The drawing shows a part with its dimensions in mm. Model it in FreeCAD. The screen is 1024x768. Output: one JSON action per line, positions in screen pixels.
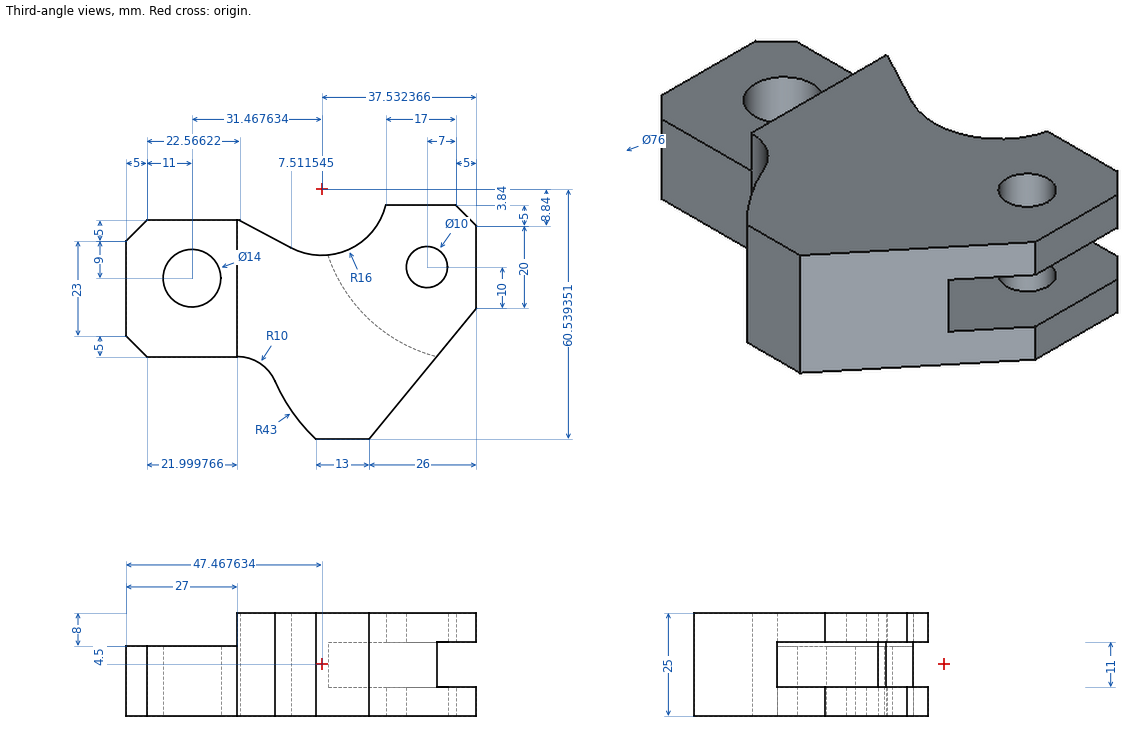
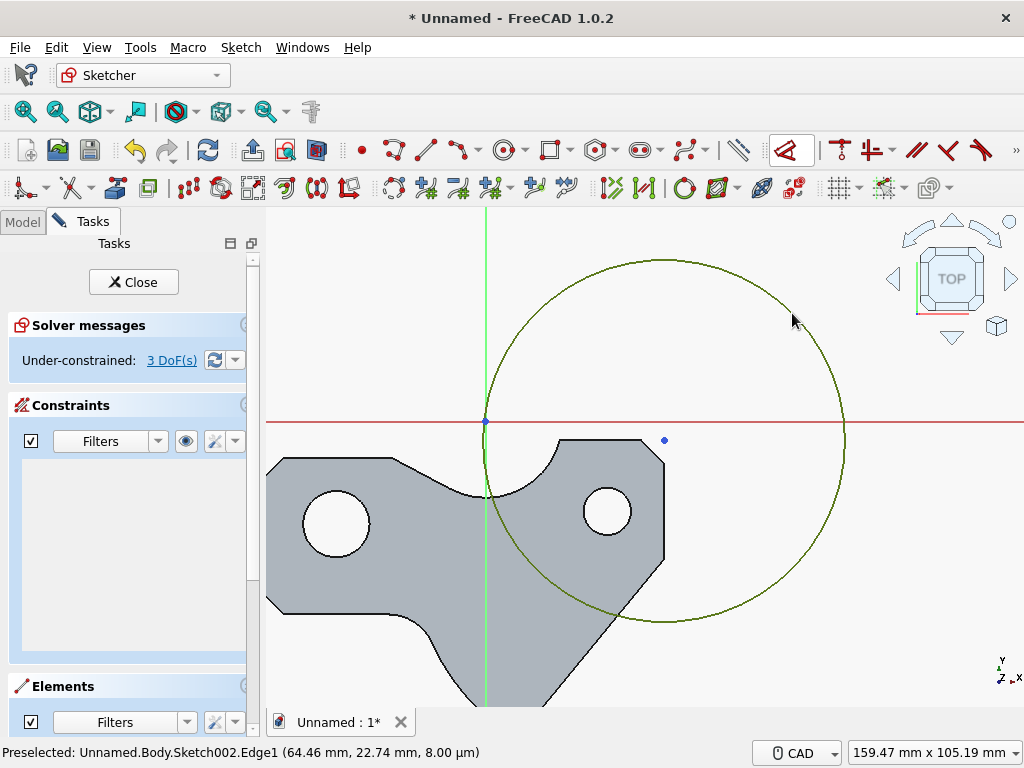
{"action": "left_click", "coordinate": [808, 150]}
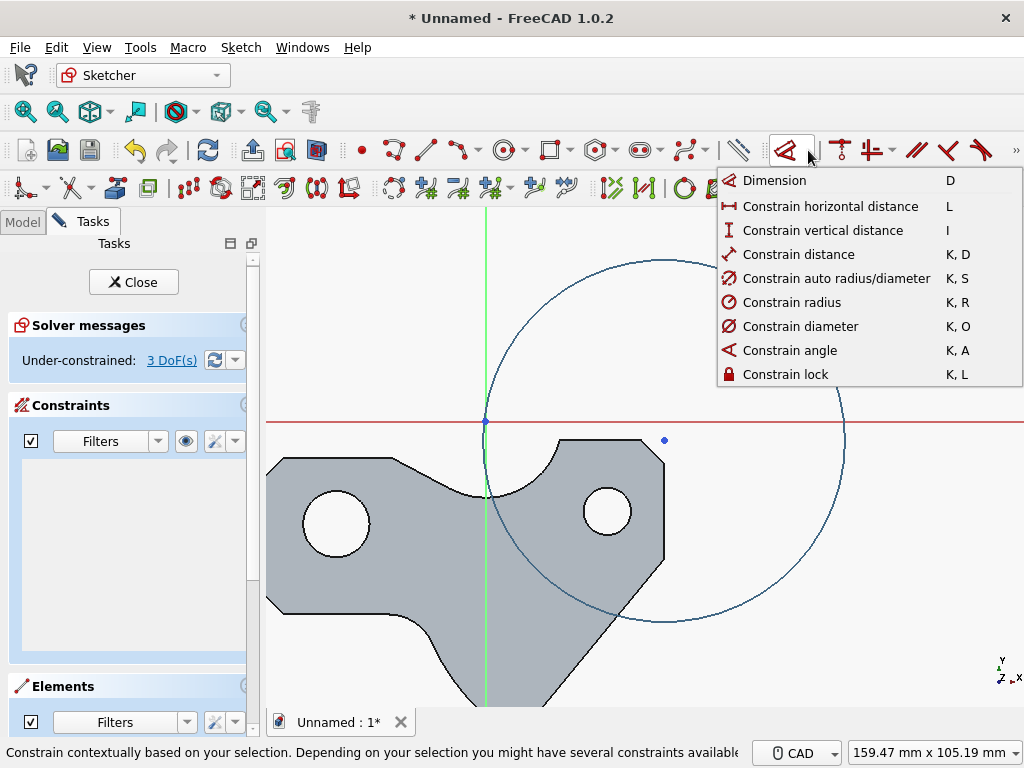
{"action": "left_click", "coordinate": [870, 326]}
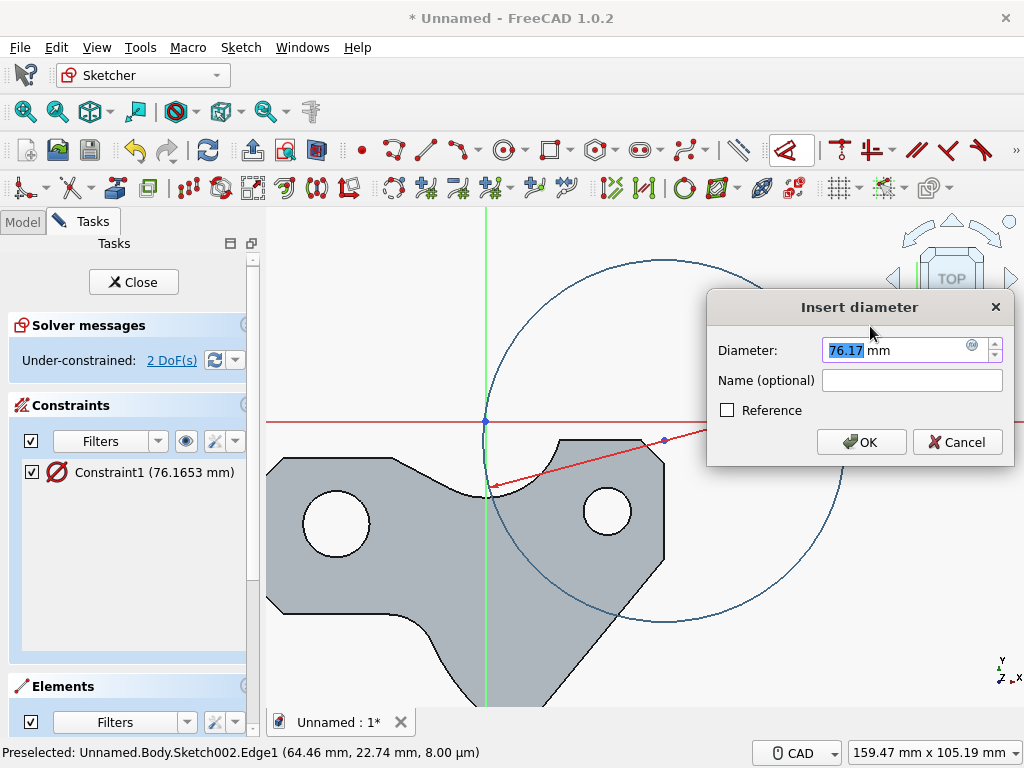
{"action": "type", "text": "76"}
{"action": "key", "text": "Return"}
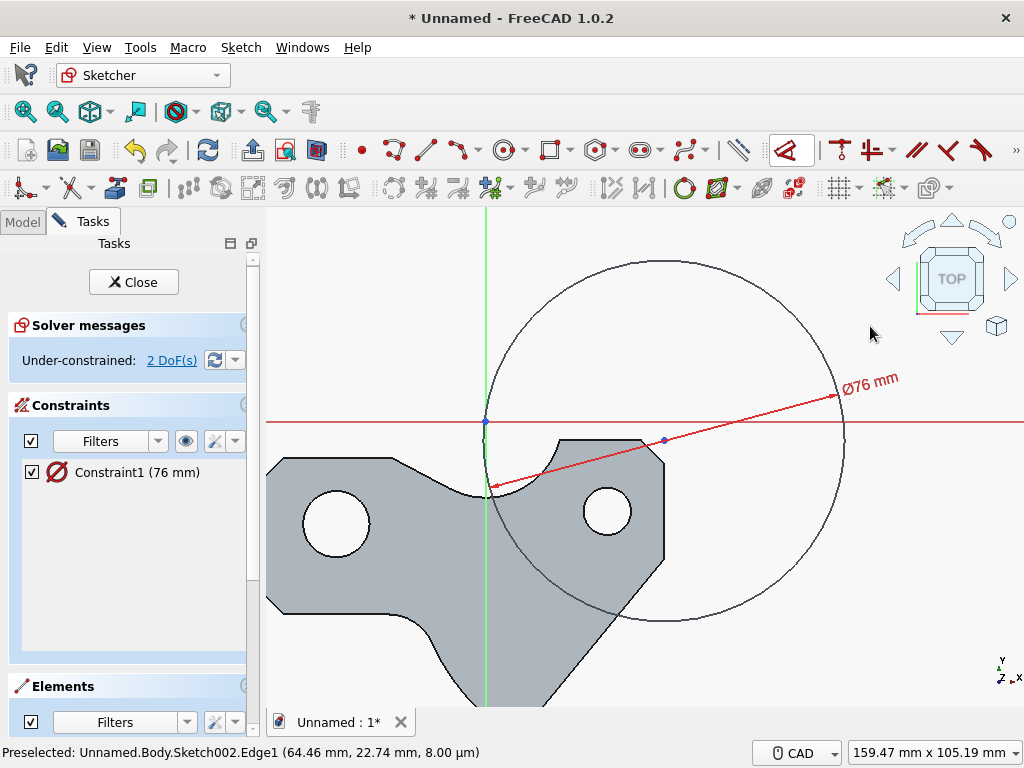
{"action": "scroll", "coordinate": [664, 441], "scroll_direction": "up", "scroll_amount": 4}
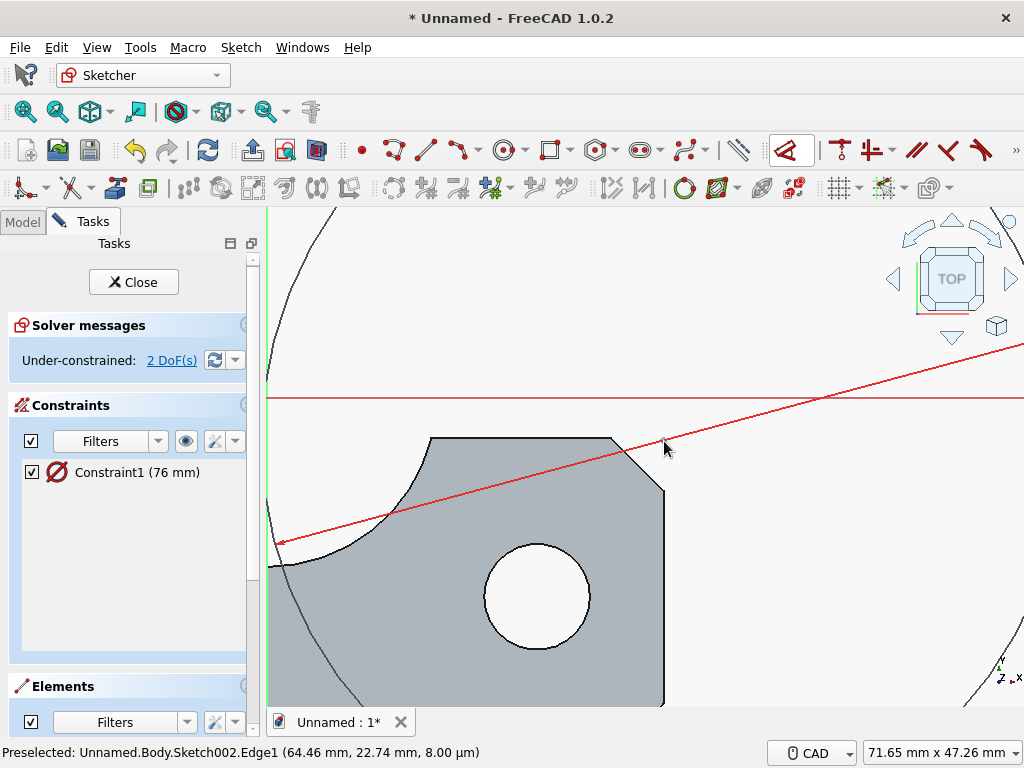
{"action": "left_click", "coordinate": [663, 440]}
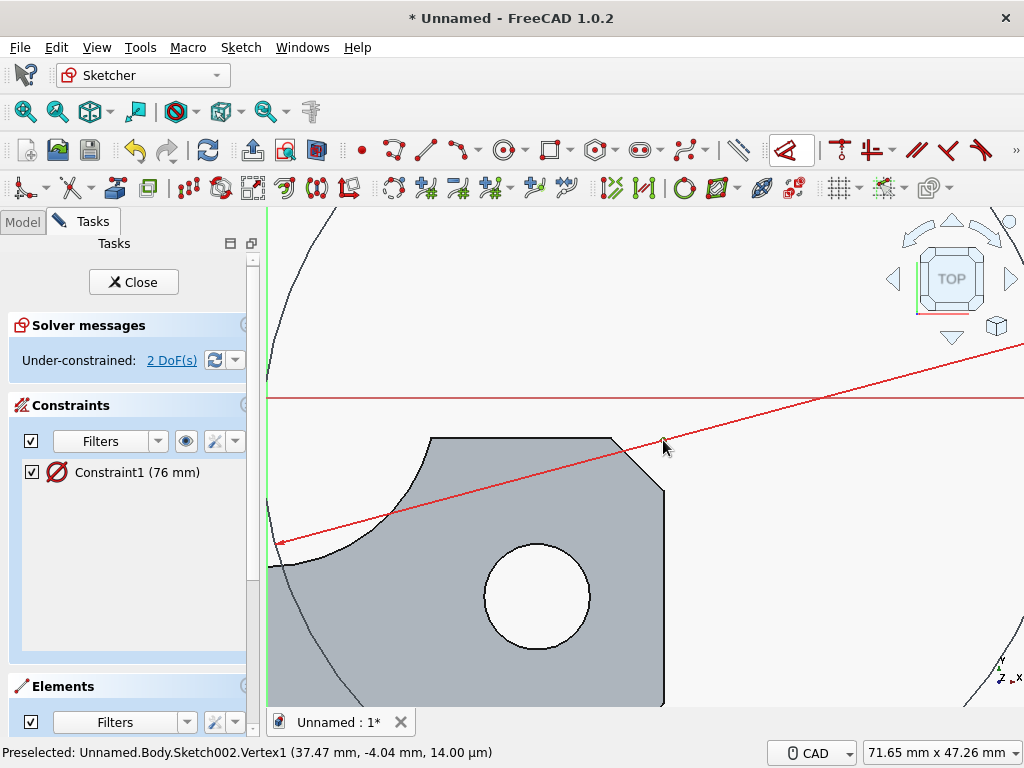
{"action": "key", "text": "i"}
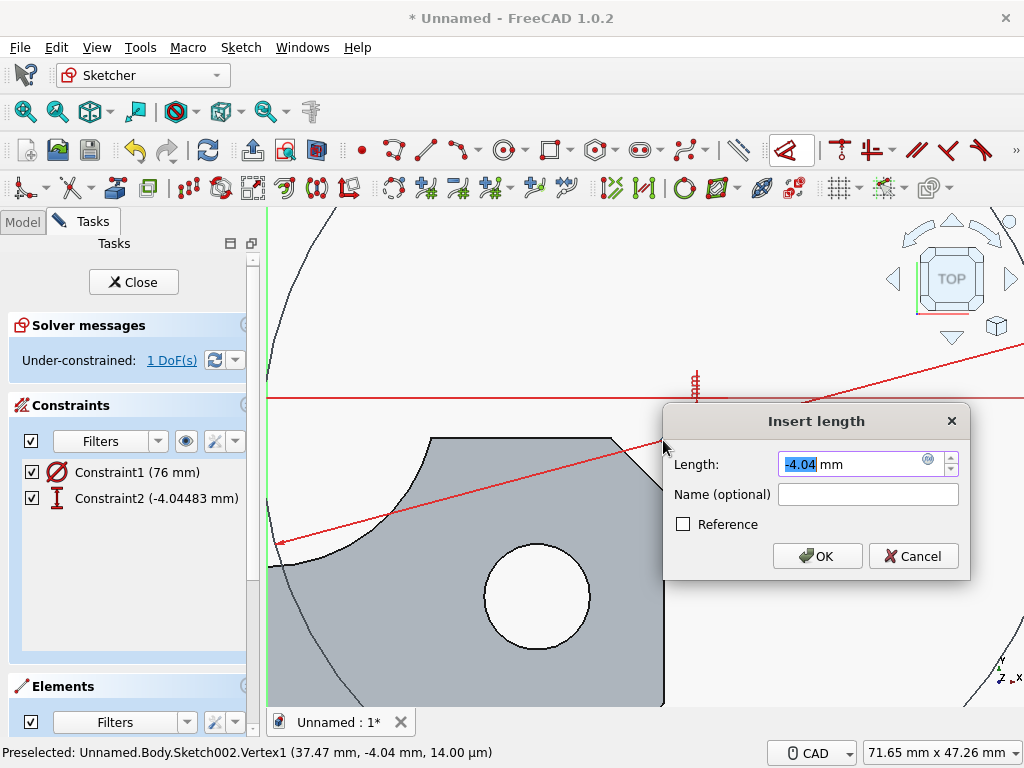
{"action": "type", "text": "-3.84"}
{"action": "key", "text": "Return"}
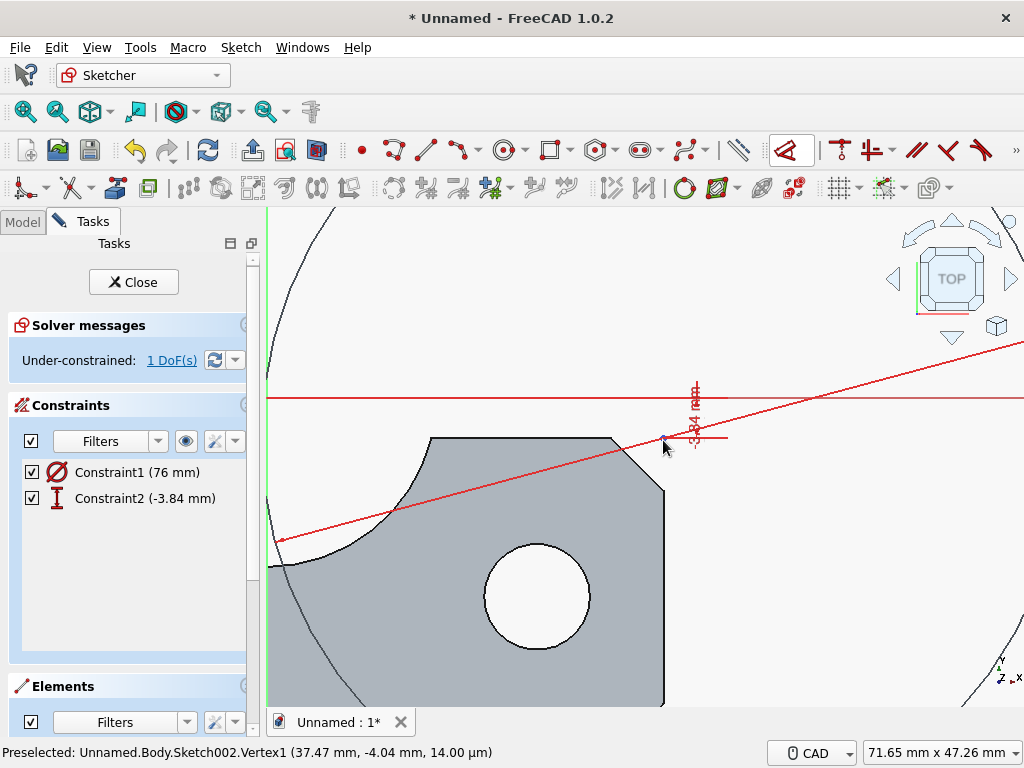
{"action": "left_click", "coordinate": [663, 438]}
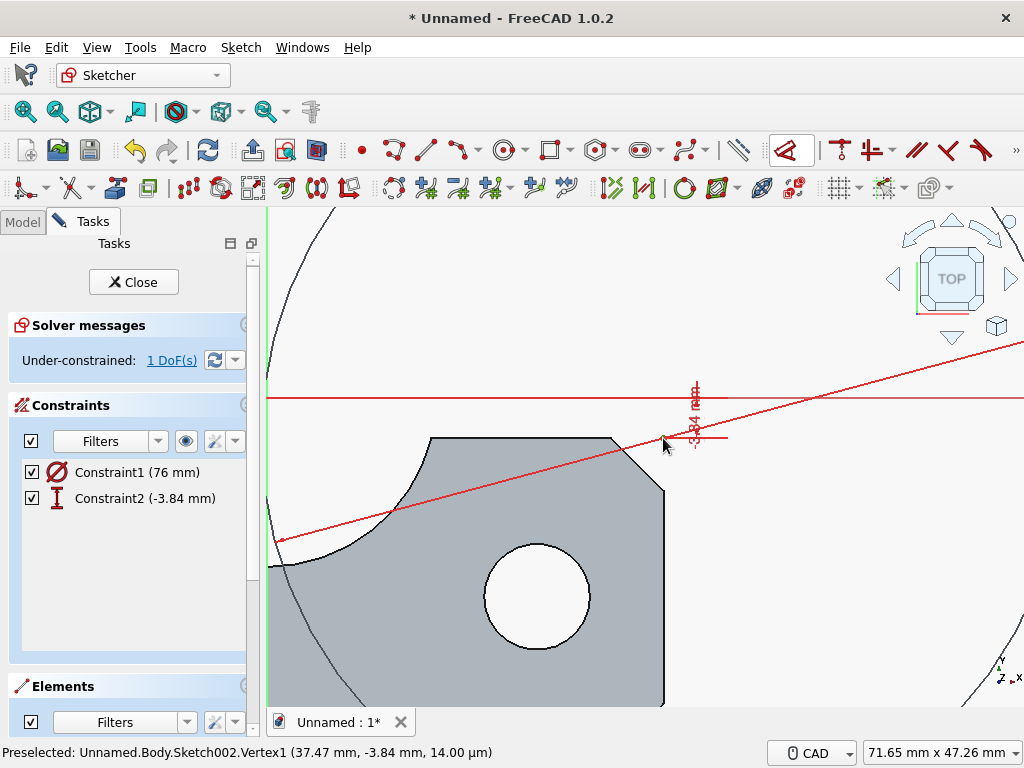
{"action": "key", "text": "l"}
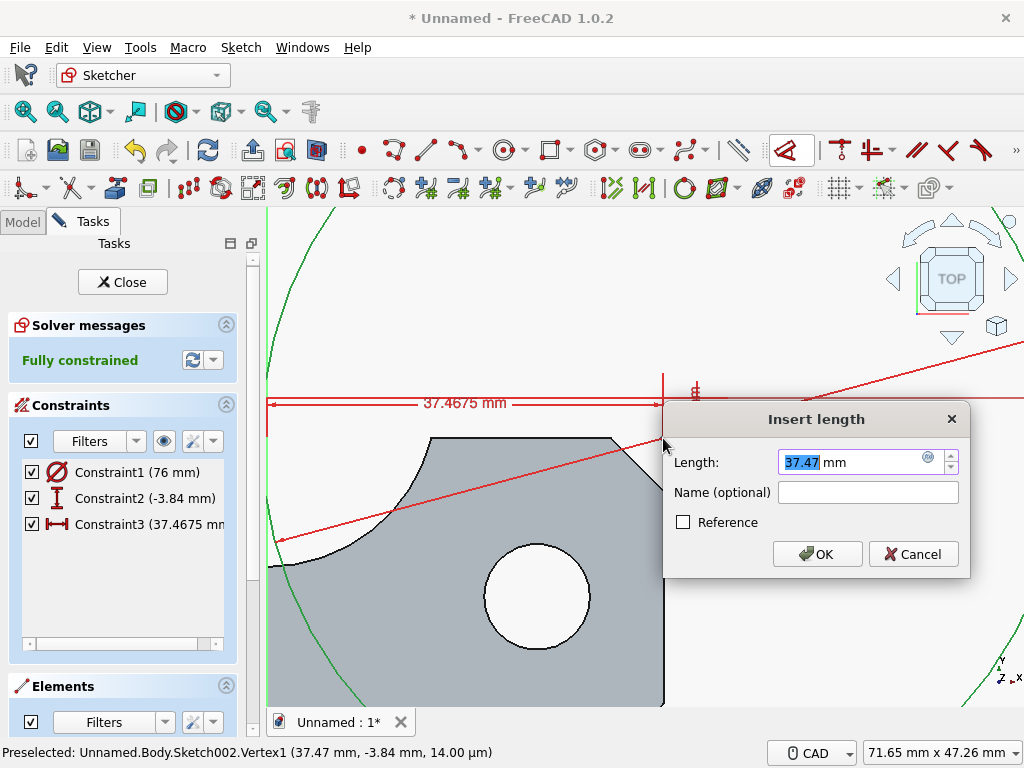
{"action": "type", "text": "37.532366"}
{"action": "key", "text": "Return"}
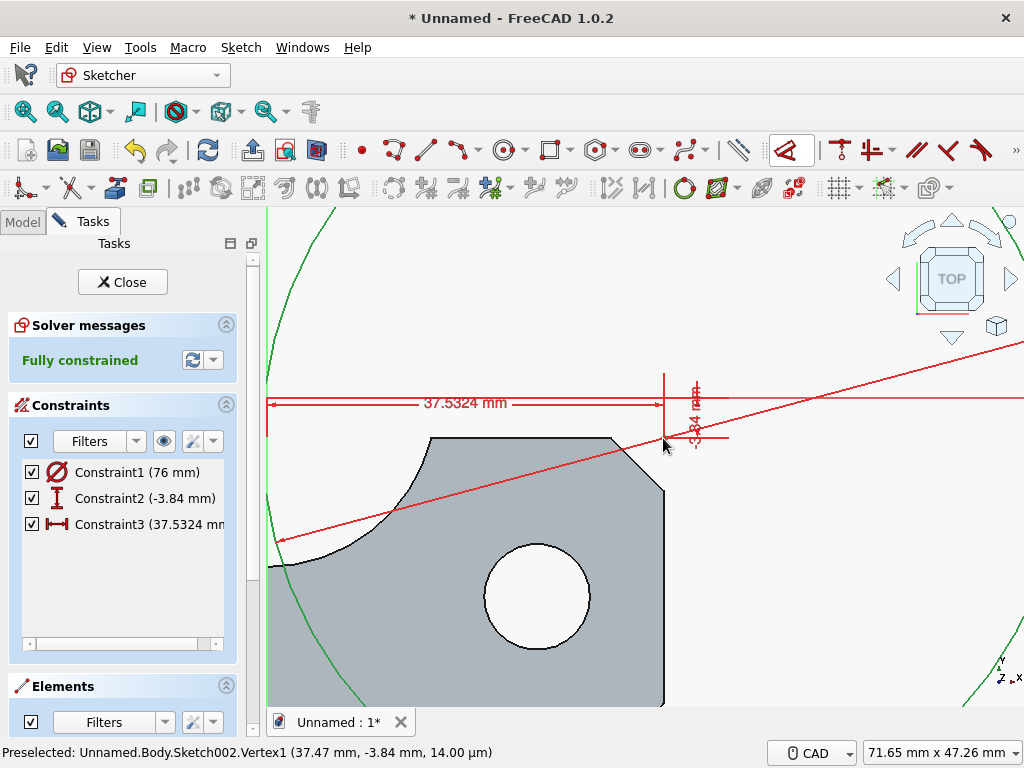
{"action": "left_click", "coordinate": [123, 282]}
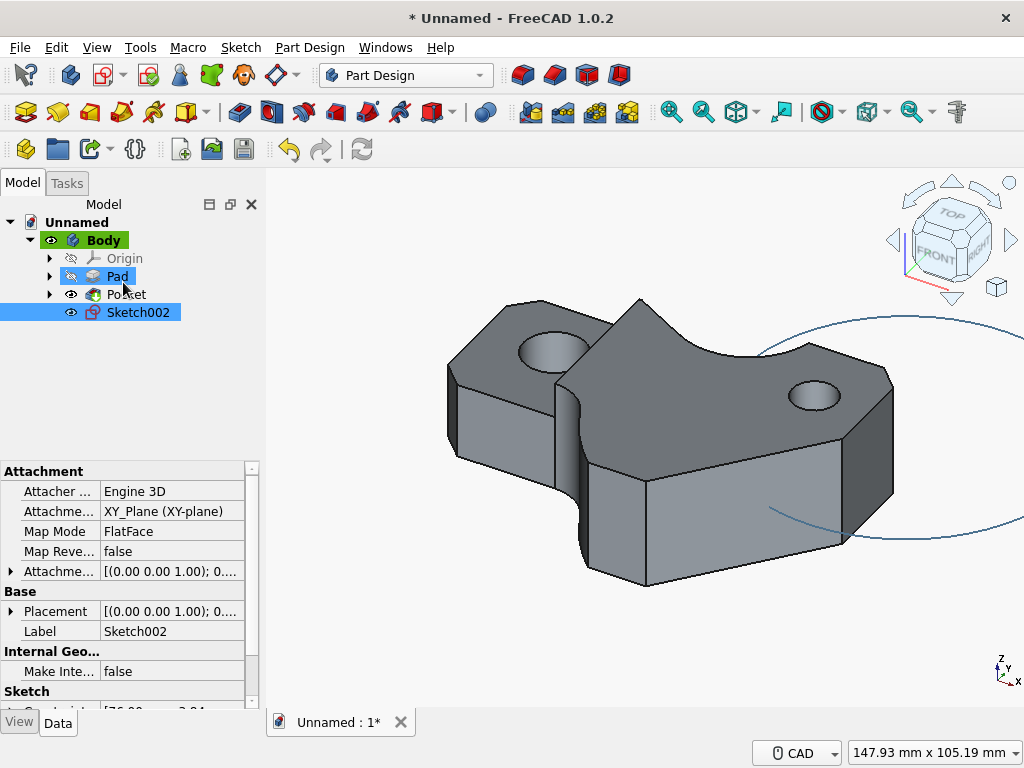
{"action": "left_click", "coordinate": [240, 112]}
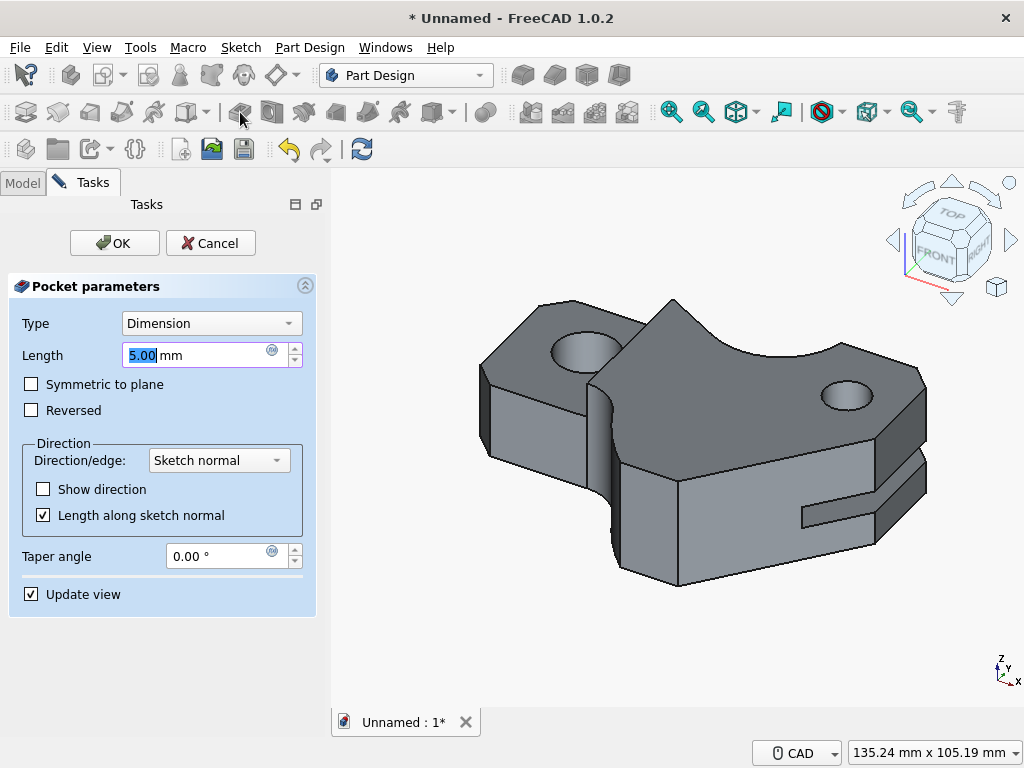
{"action": "type", "text": "11"}
{"action": "key", "text": "Tab"}